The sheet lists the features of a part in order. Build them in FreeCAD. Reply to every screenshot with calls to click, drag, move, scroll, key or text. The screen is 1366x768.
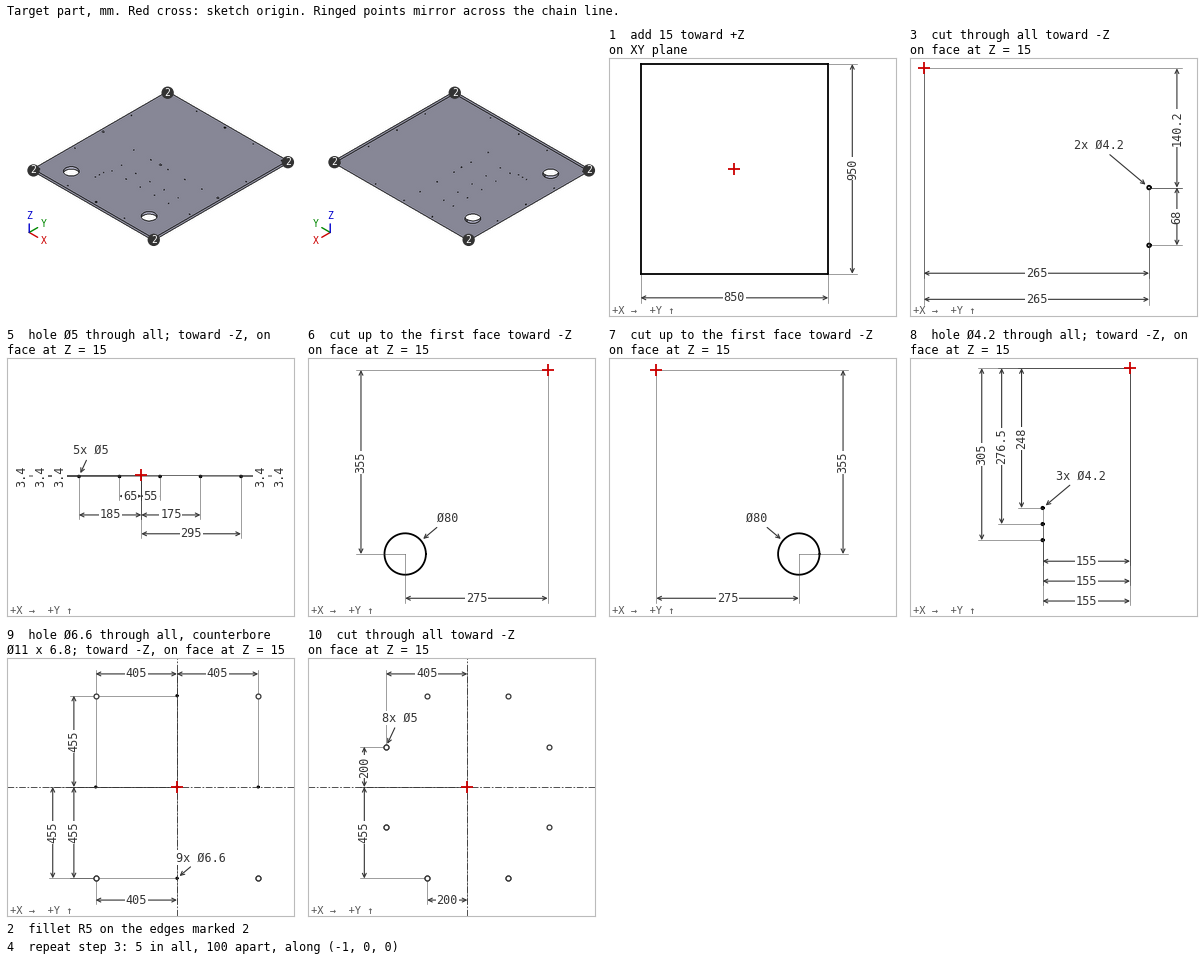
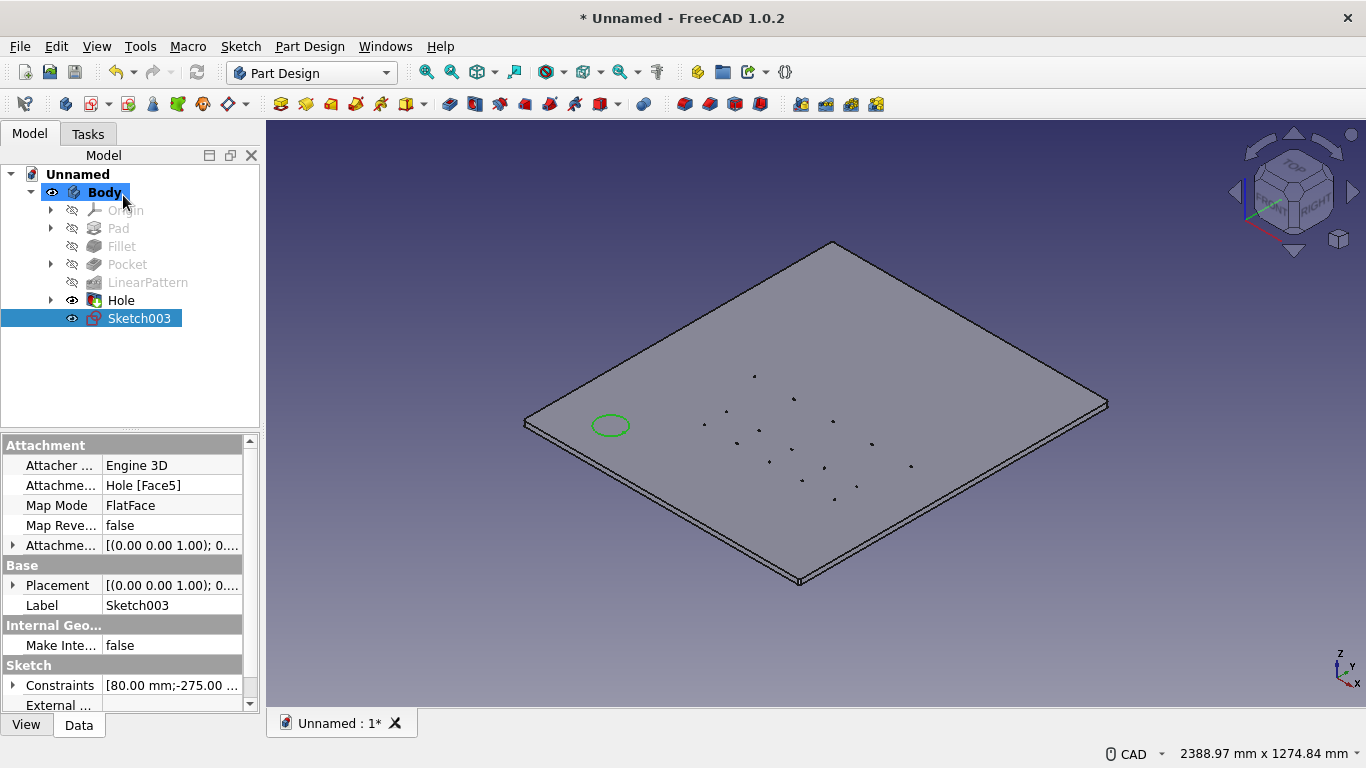
click(450, 104)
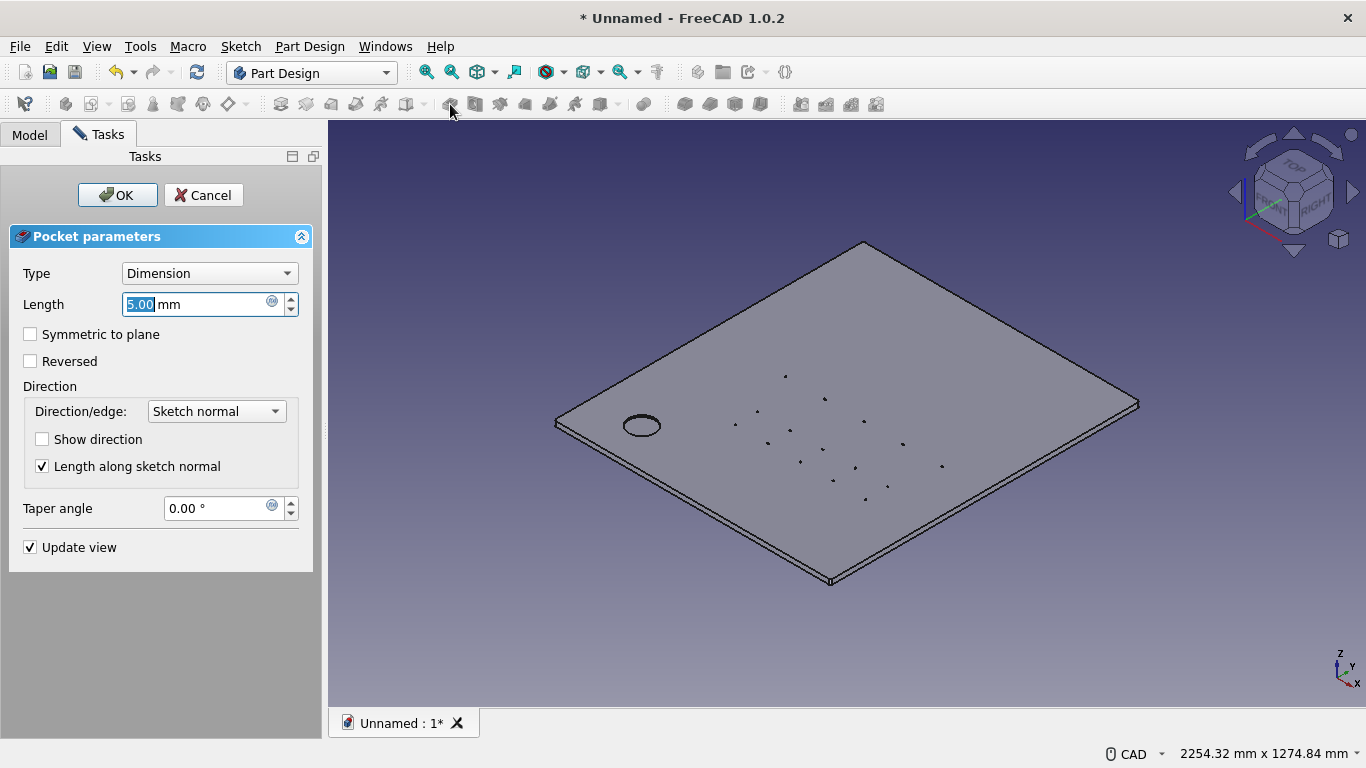
click(210, 274)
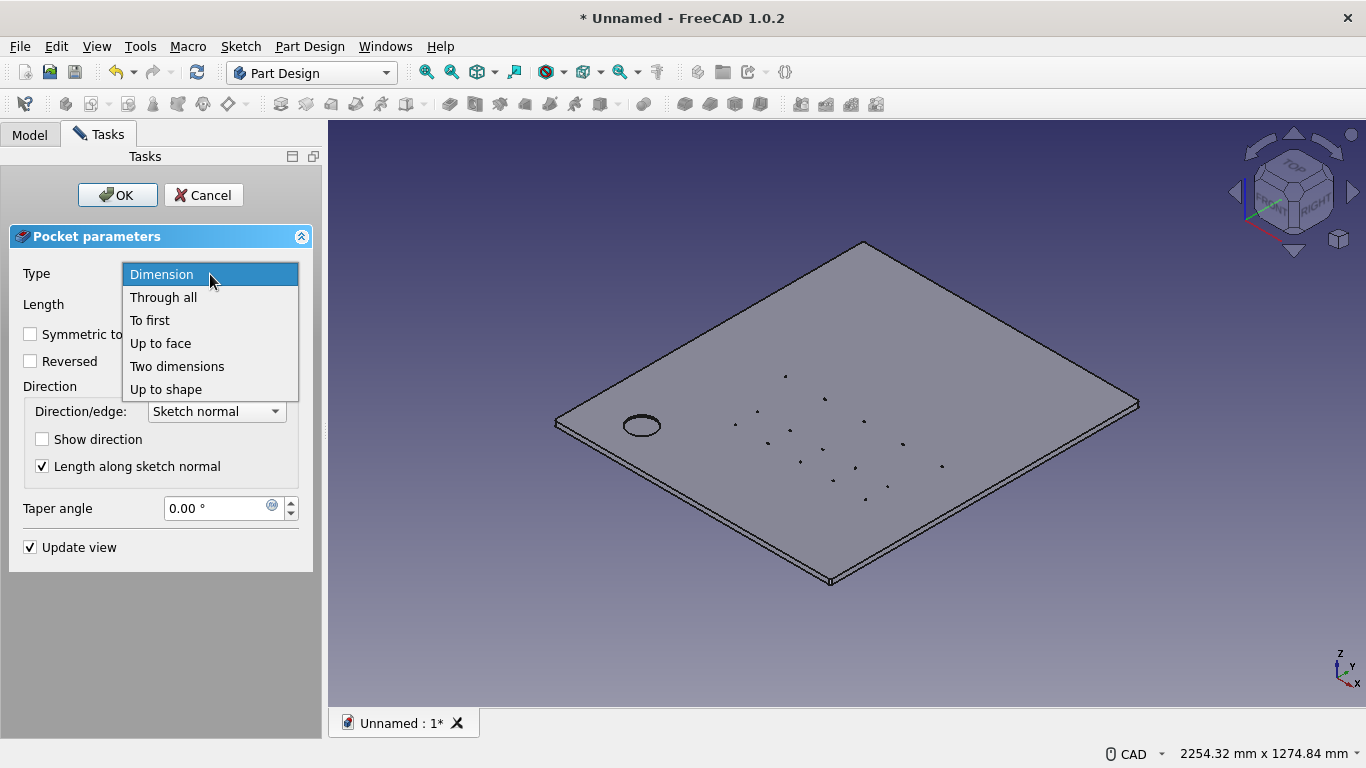
click(208, 320)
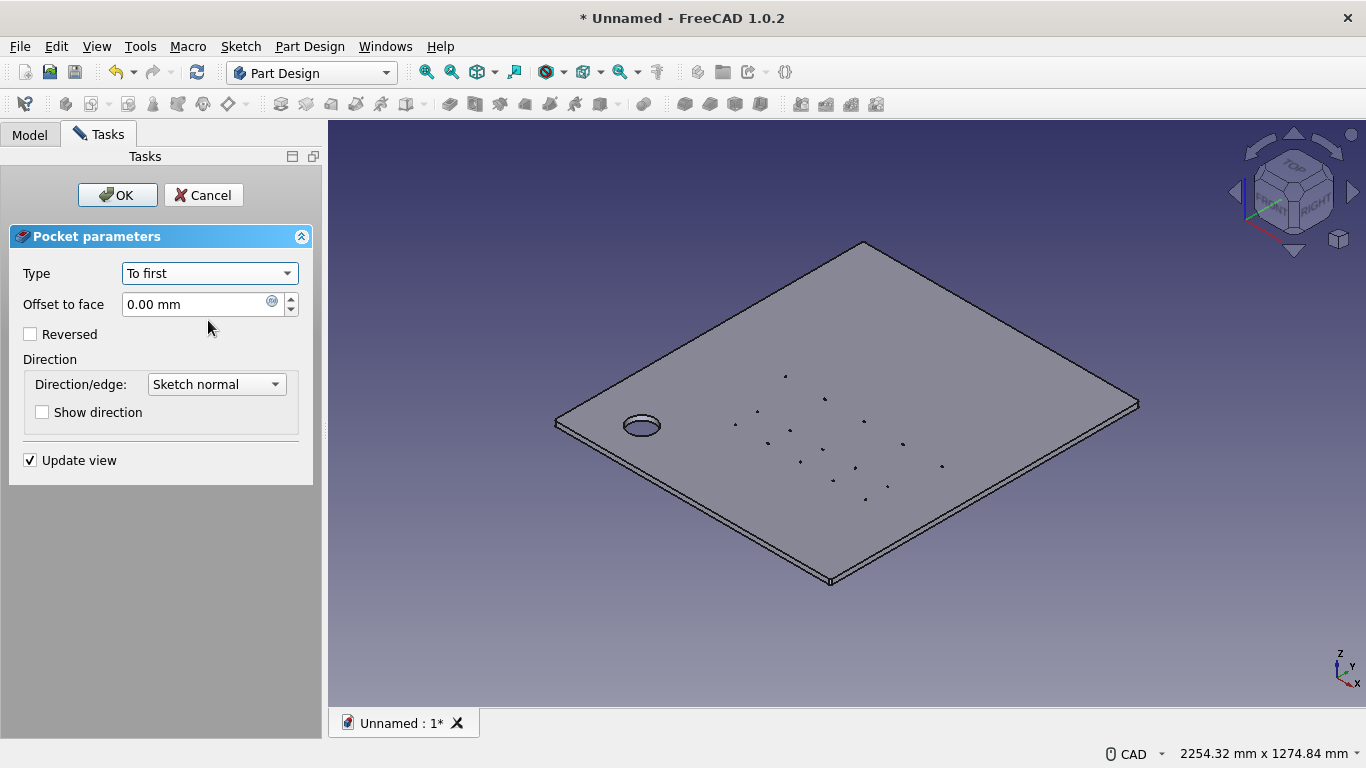
click(118, 195)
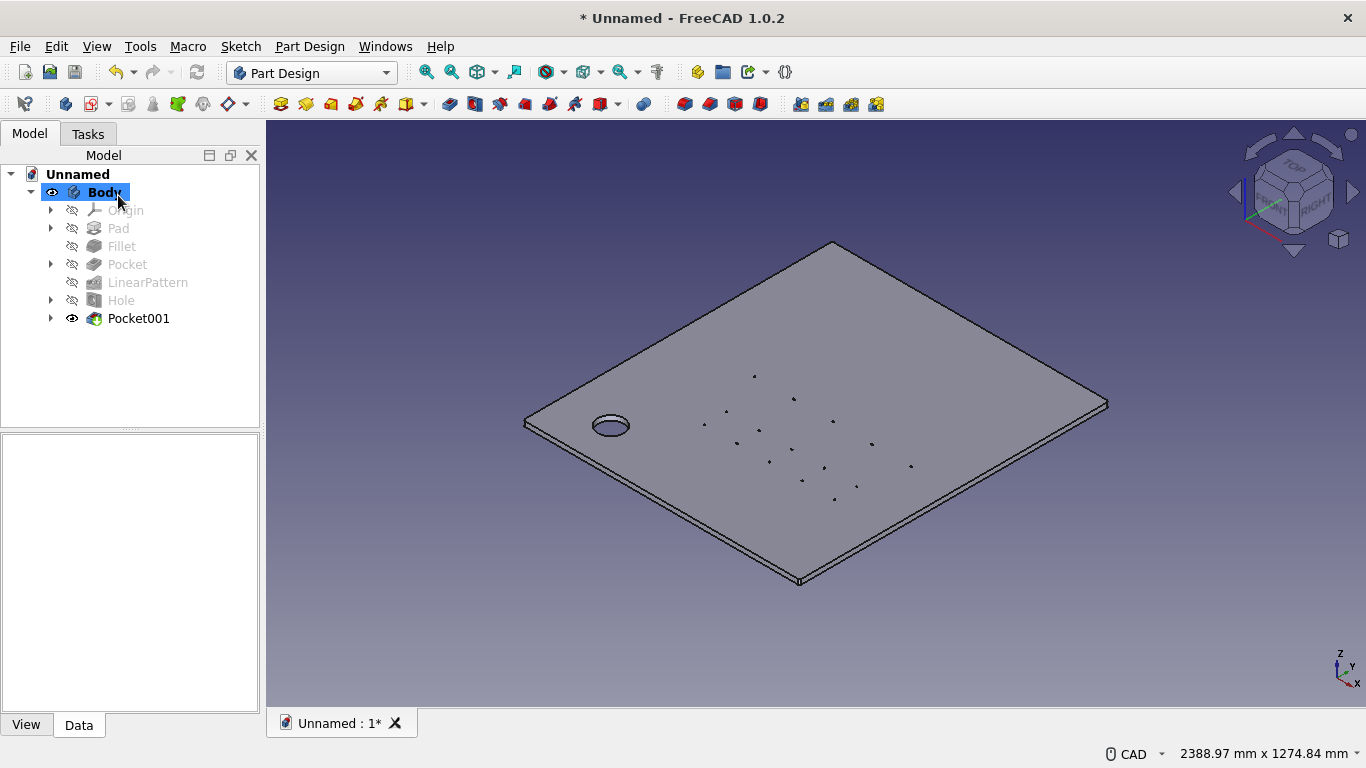
click(944, 381)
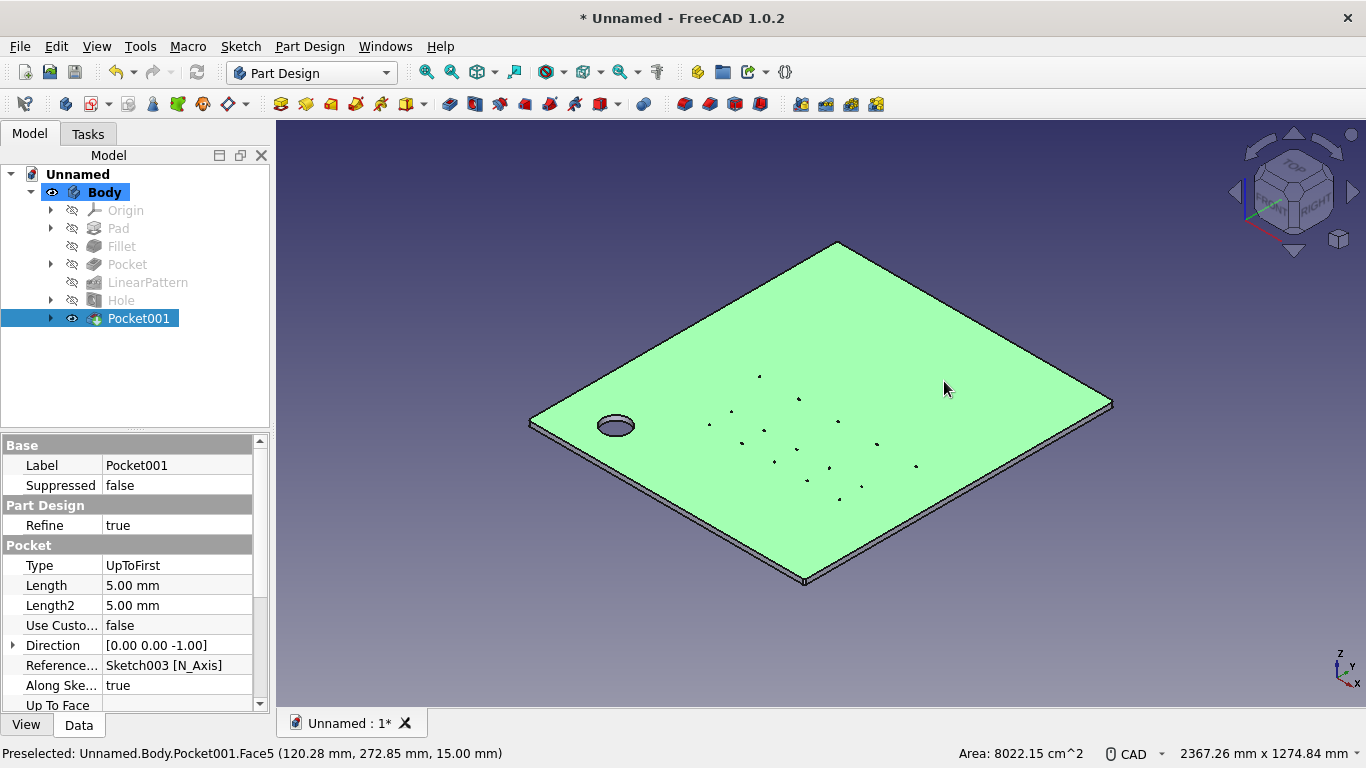
click(90, 104)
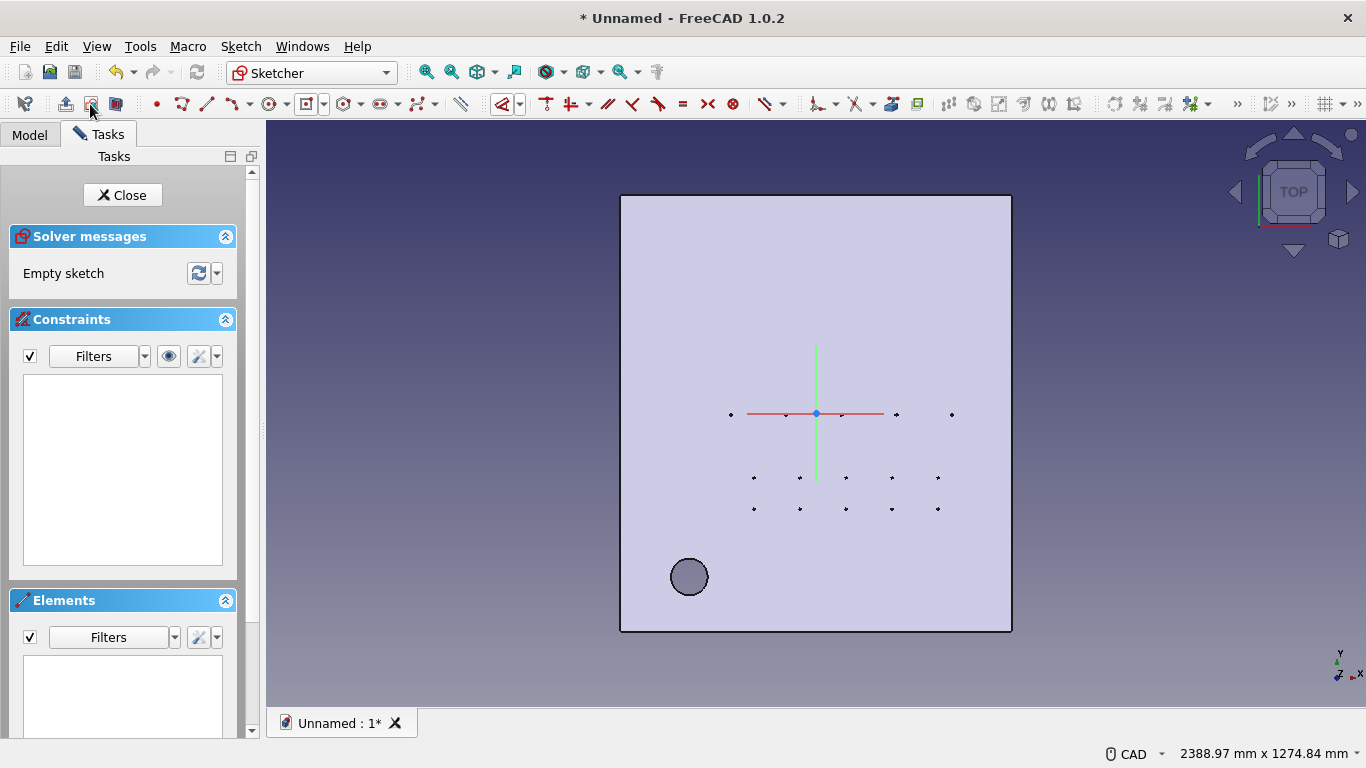
scroll(962, 593, up, 12)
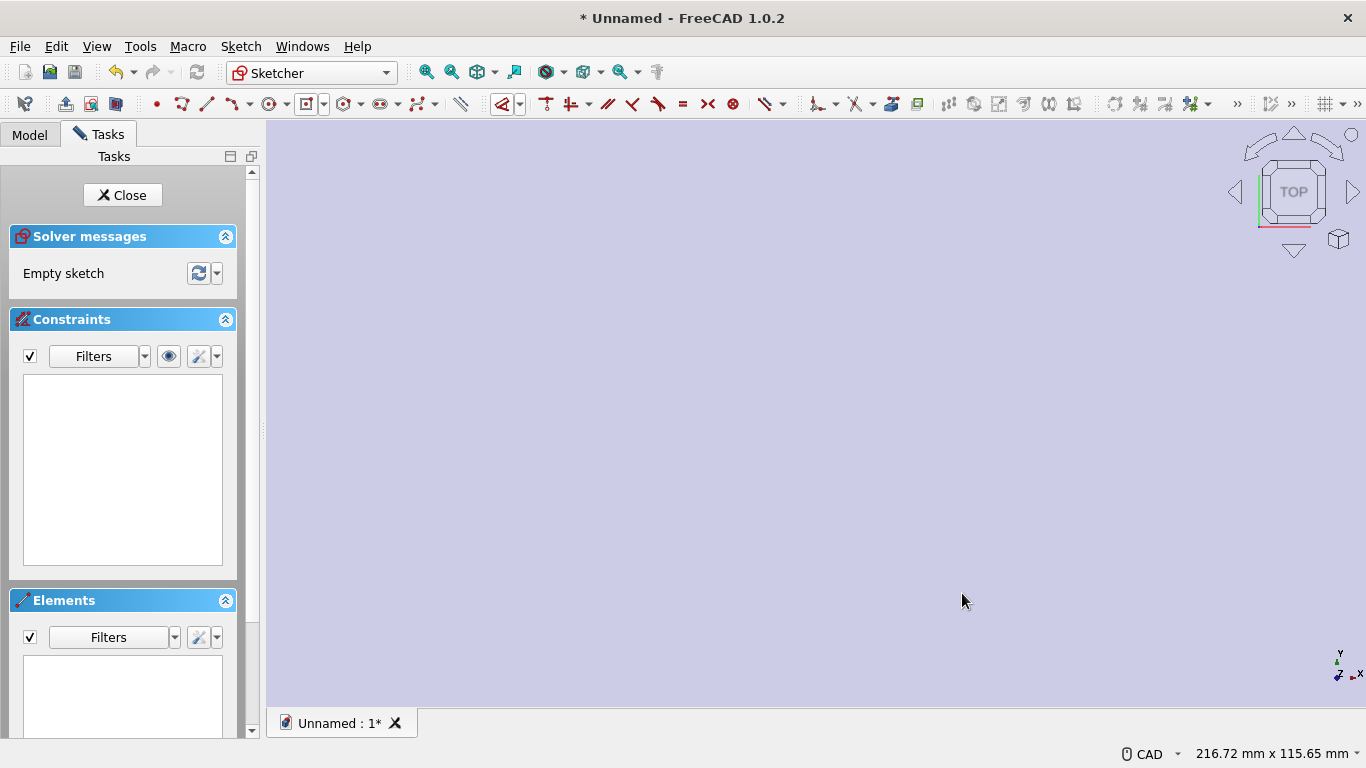
click(268, 104)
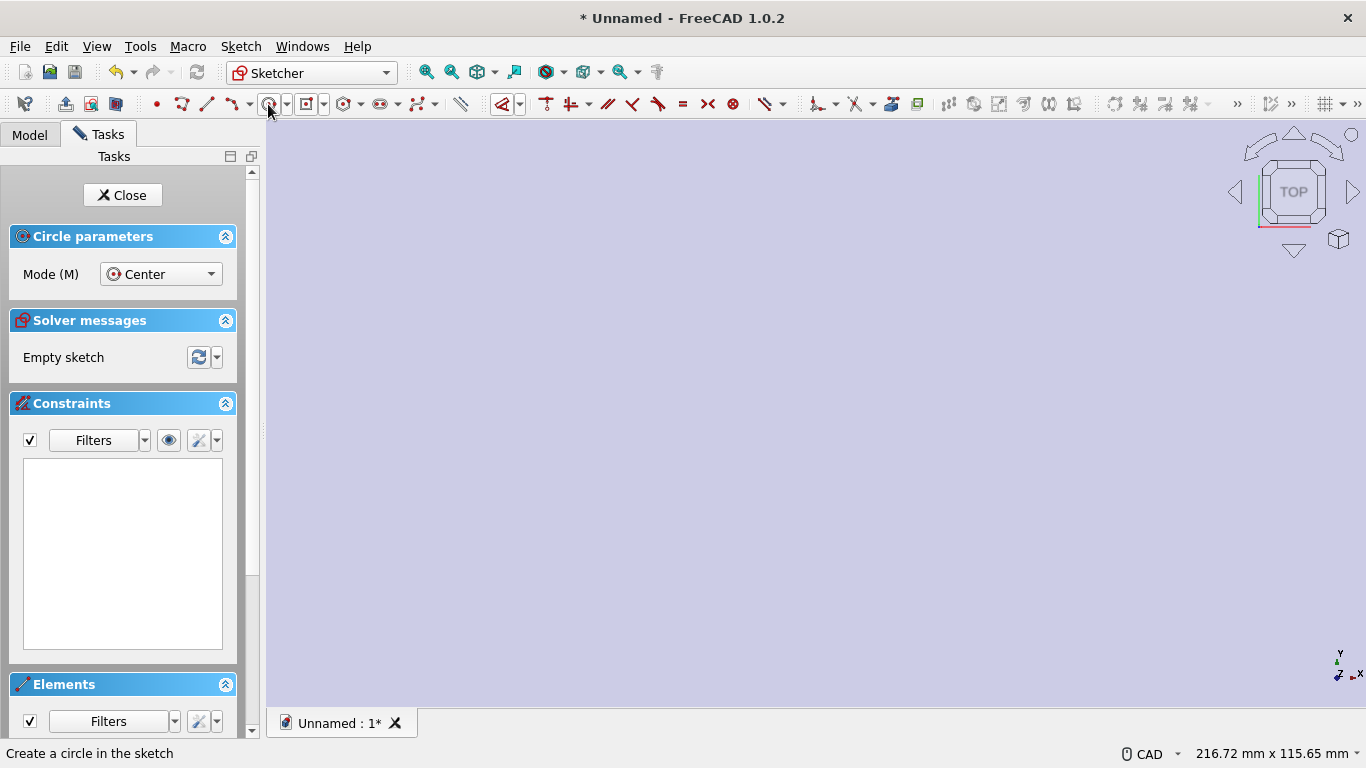
click(742, 408)
move(886, 265)